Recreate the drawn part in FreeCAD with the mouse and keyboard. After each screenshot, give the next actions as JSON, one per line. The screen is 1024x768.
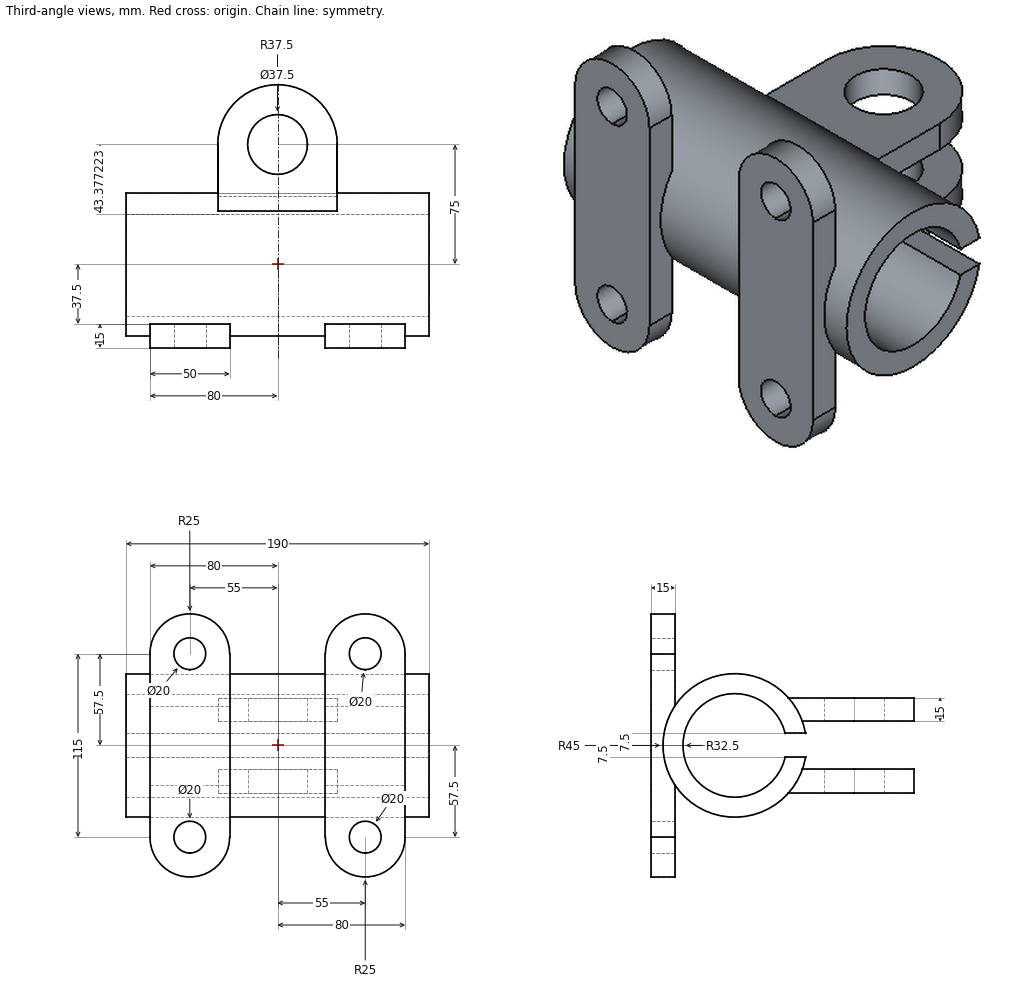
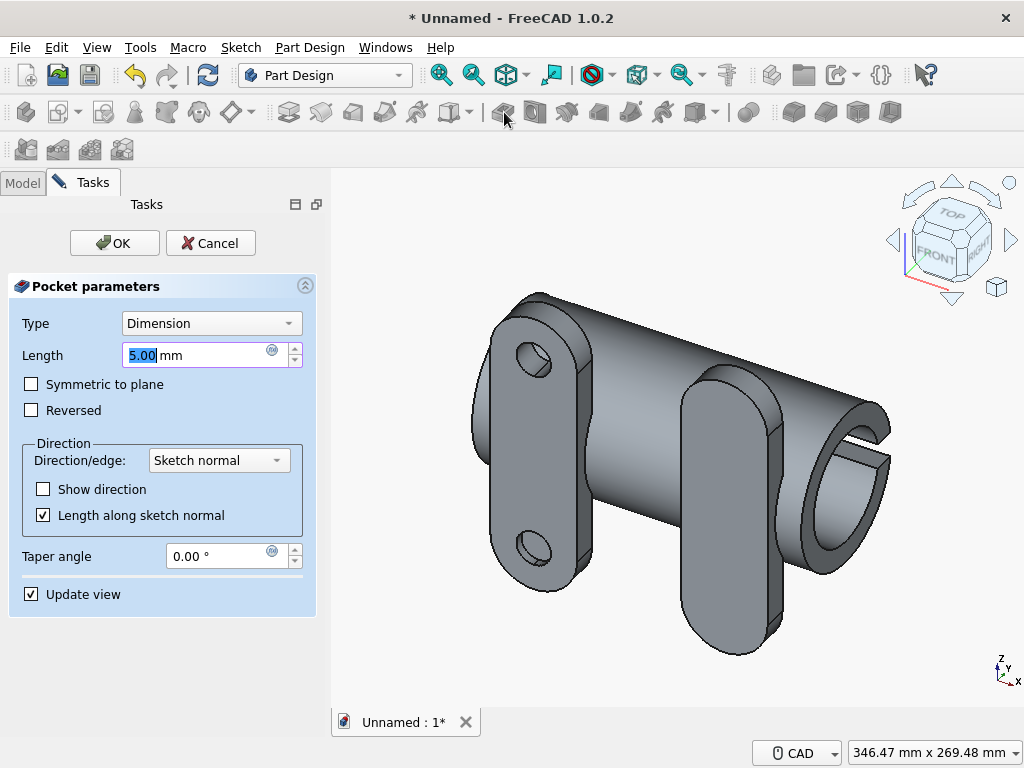
{"action": "left_click", "coordinate": [212, 324]}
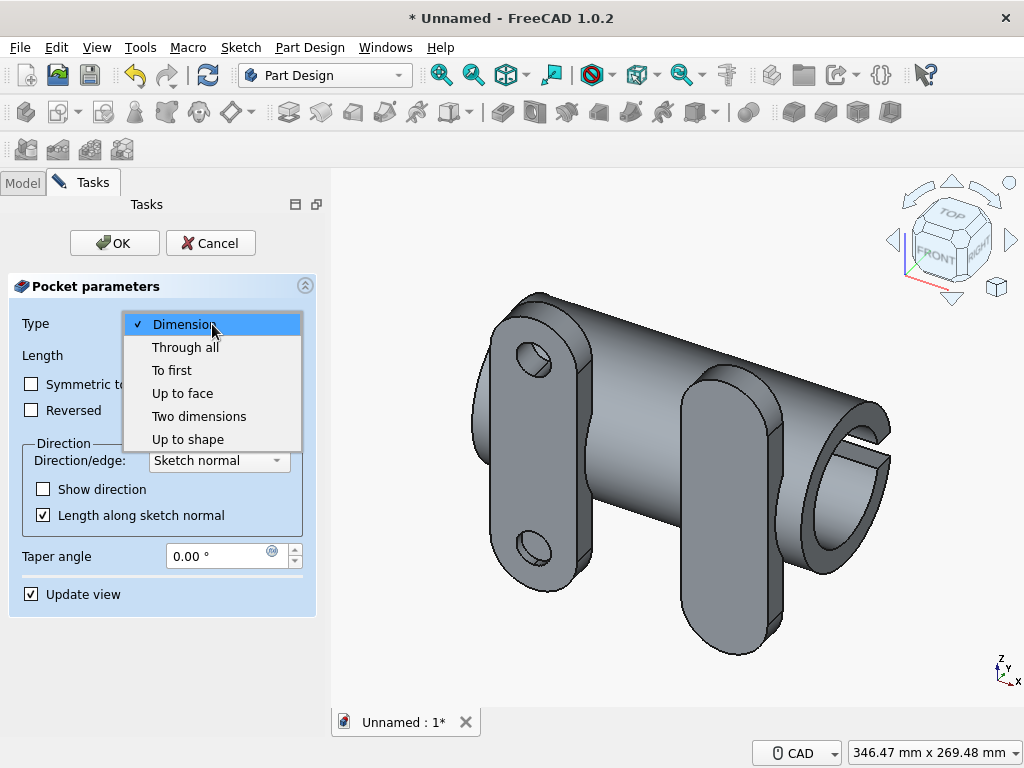
{"action": "left_click", "coordinate": [212, 370]}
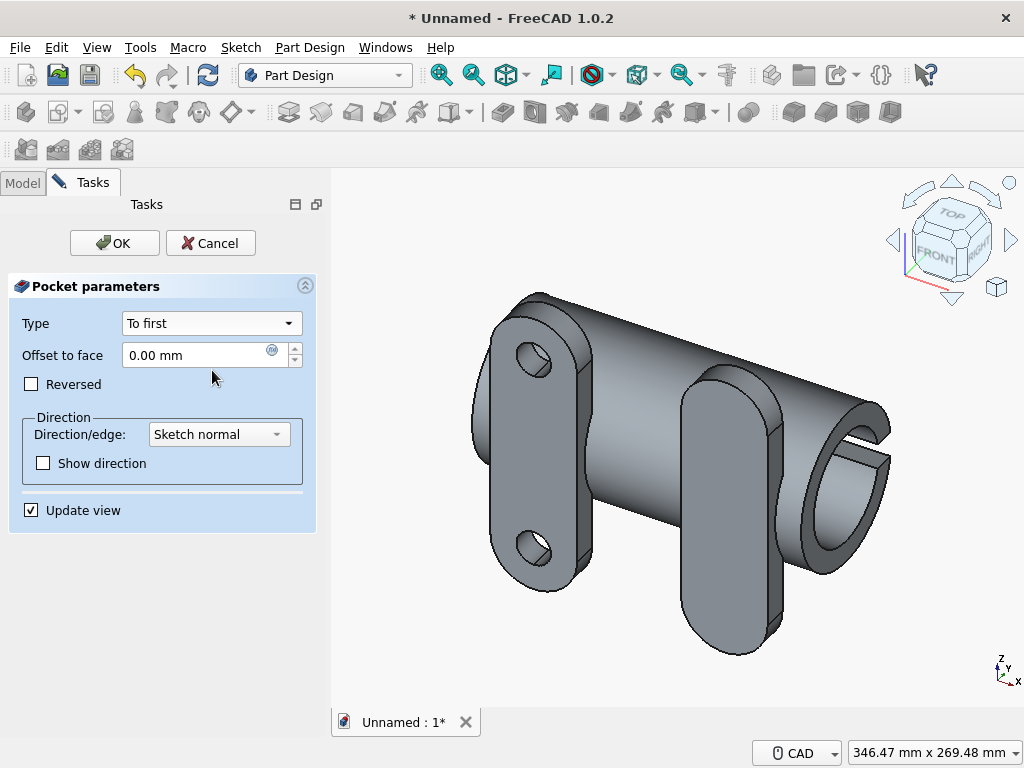
{"action": "left_click", "coordinate": [115, 243]}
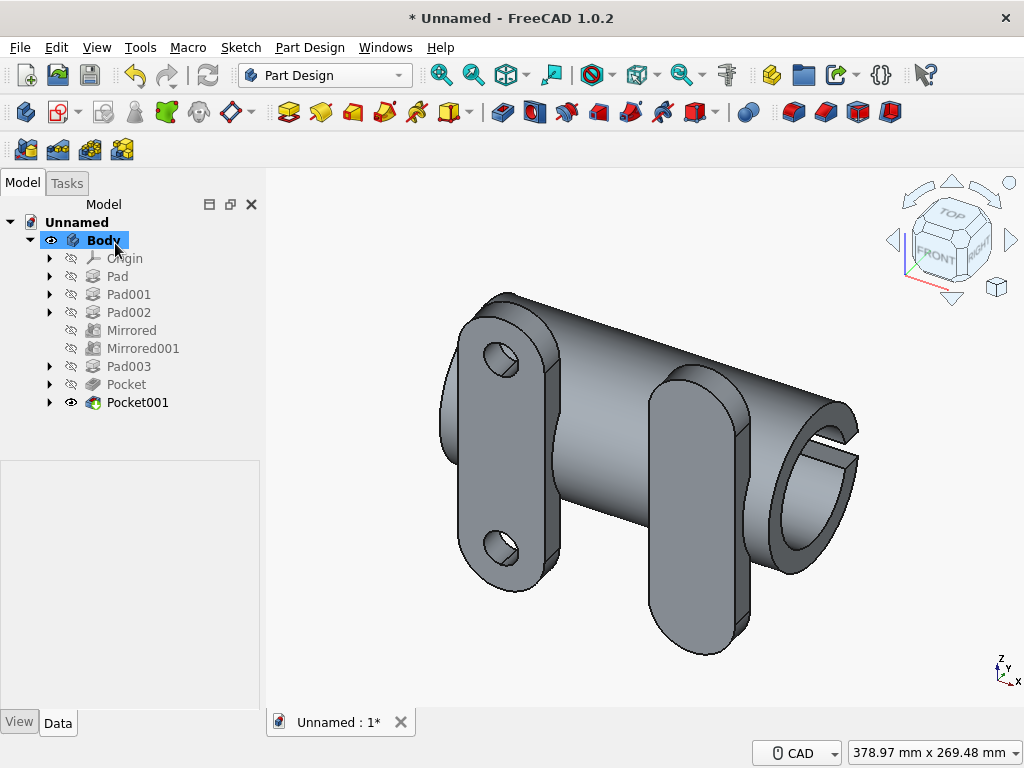
{"action": "left_click", "coordinate": [692, 516]}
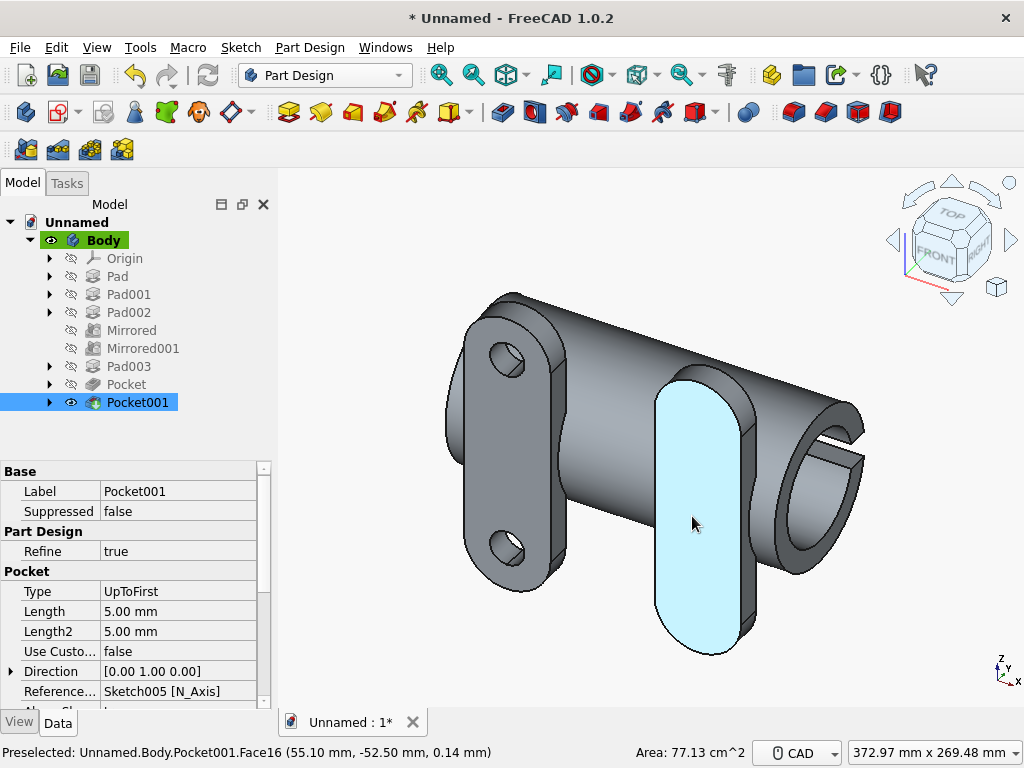
{"action": "left_click", "coordinate": [58, 112]}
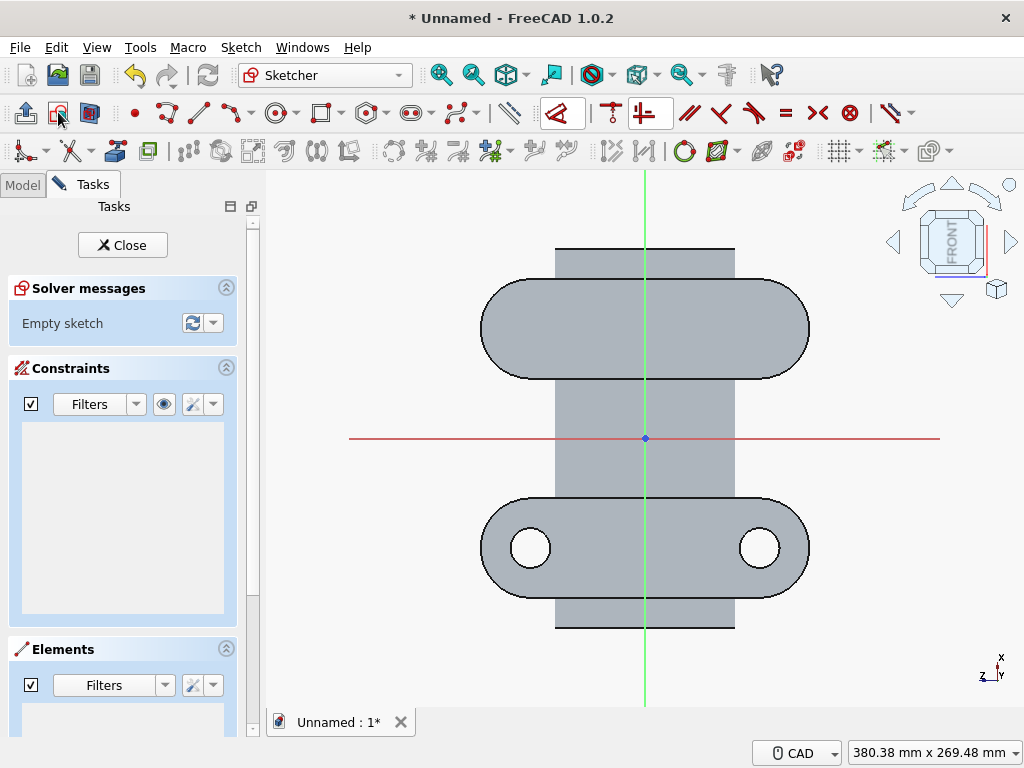
{"action": "scroll", "coordinate": [782, 315], "scroll_direction": "up", "scroll_amount": 11}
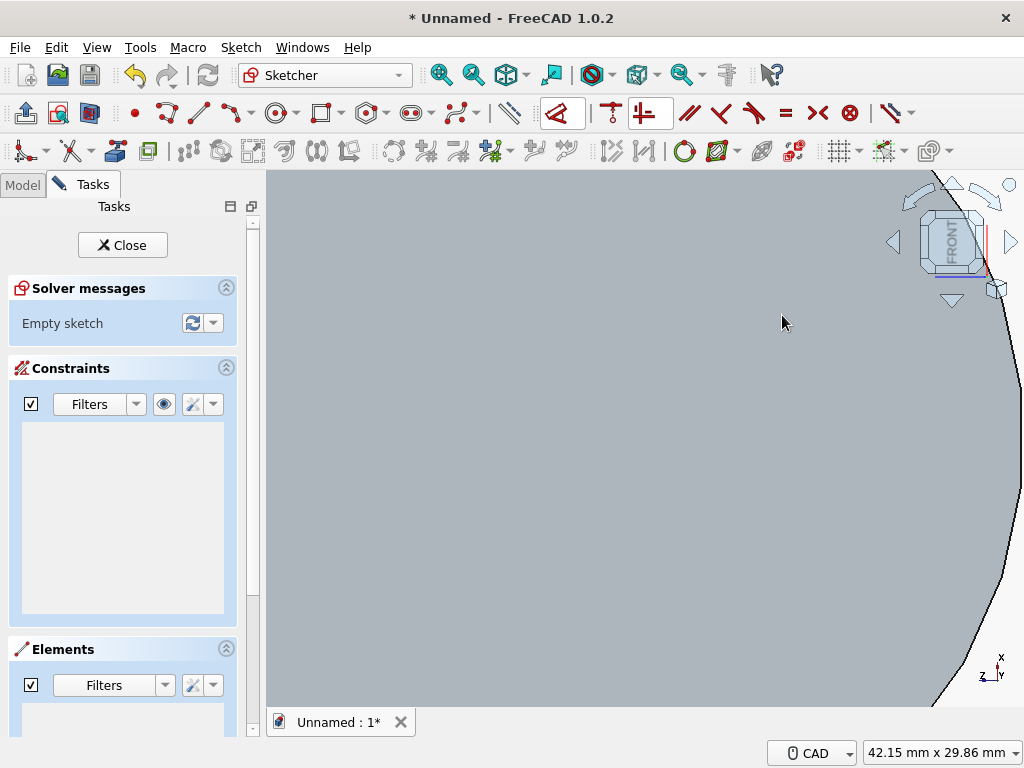
{"action": "left_click", "coordinate": [276, 114]}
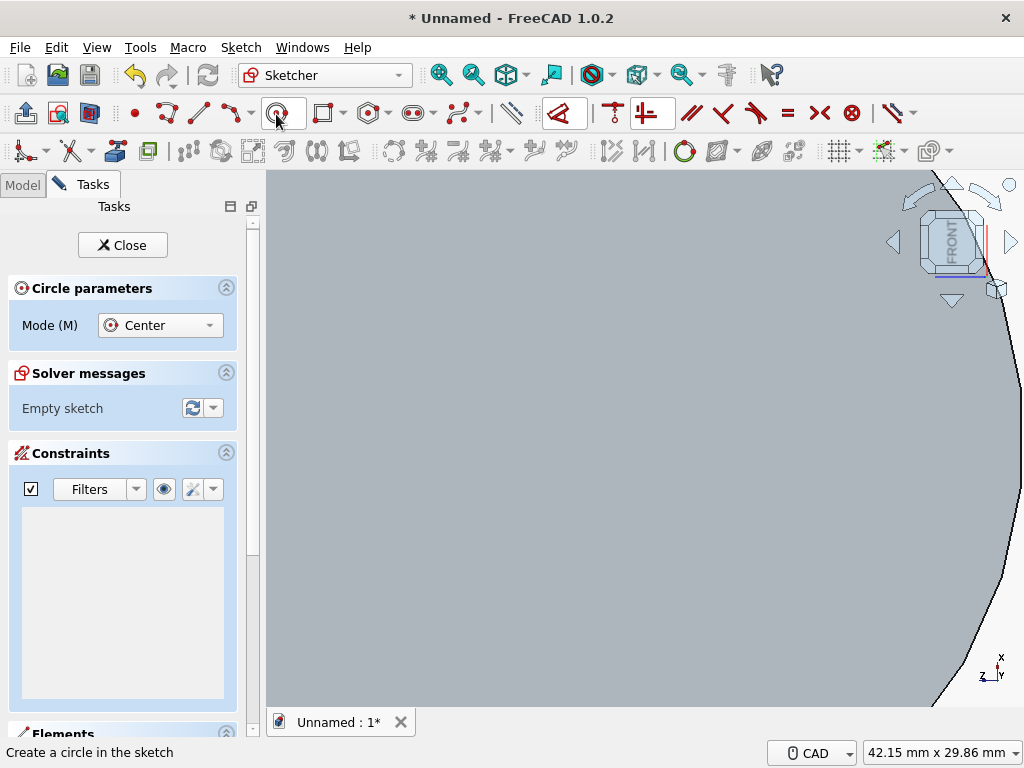
{"action": "left_click", "coordinate": [574, 438]}
{"action": "left_click", "coordinate": [701, 311]}
{"action": "key", "text": "Escape"}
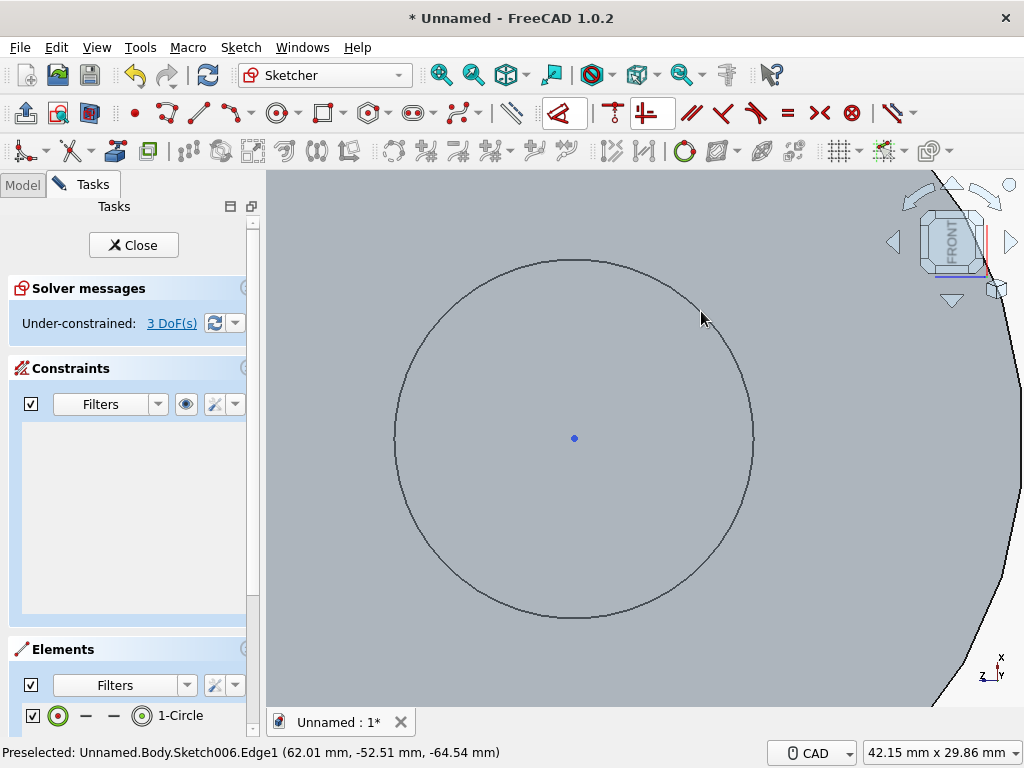
{"action": "left_click", "coordinate": [701, 312]}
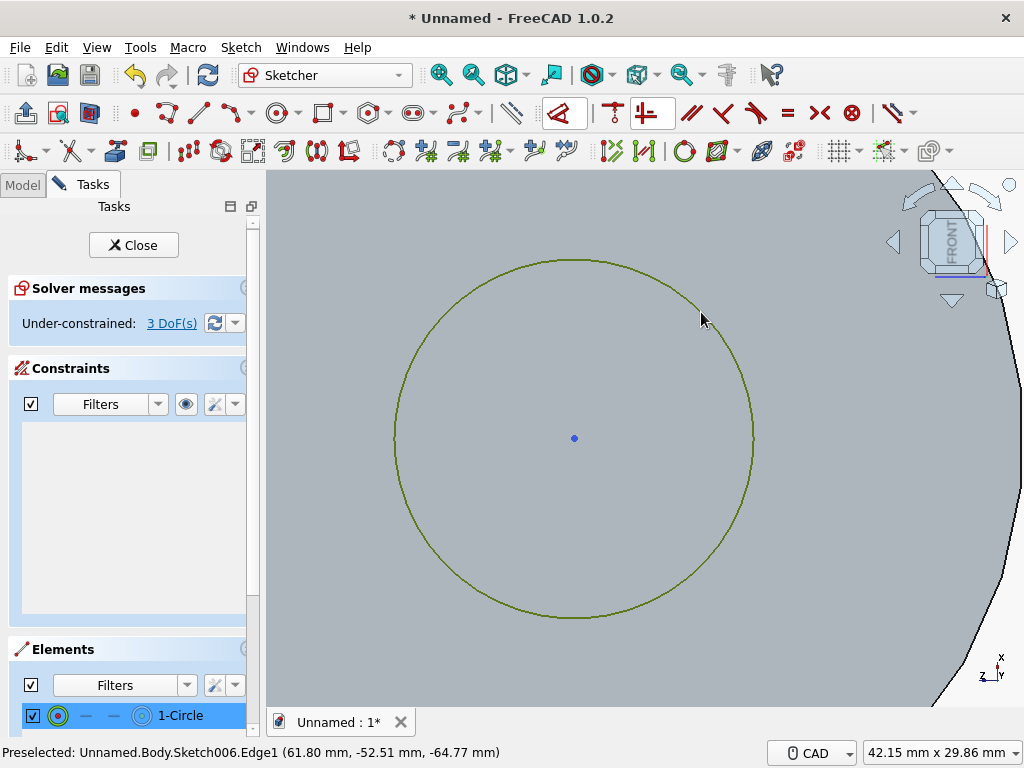
{"action": "left_click", "coordinate": [582, 114]}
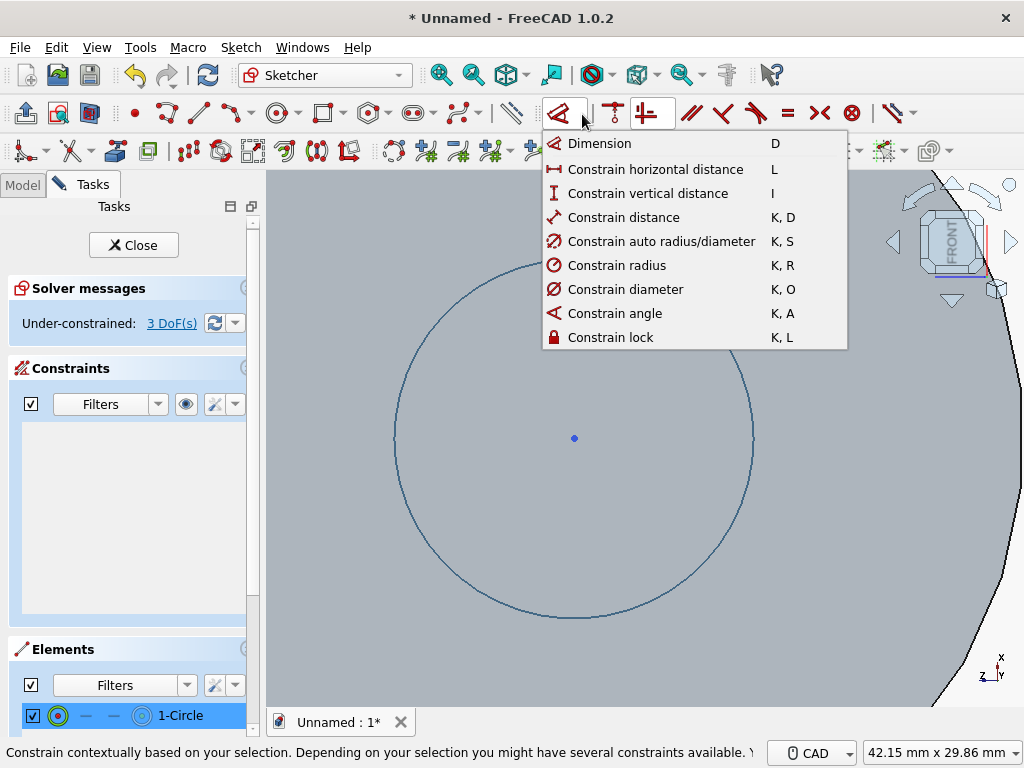
{"action": "left_click", "coordinate": [695, 289]}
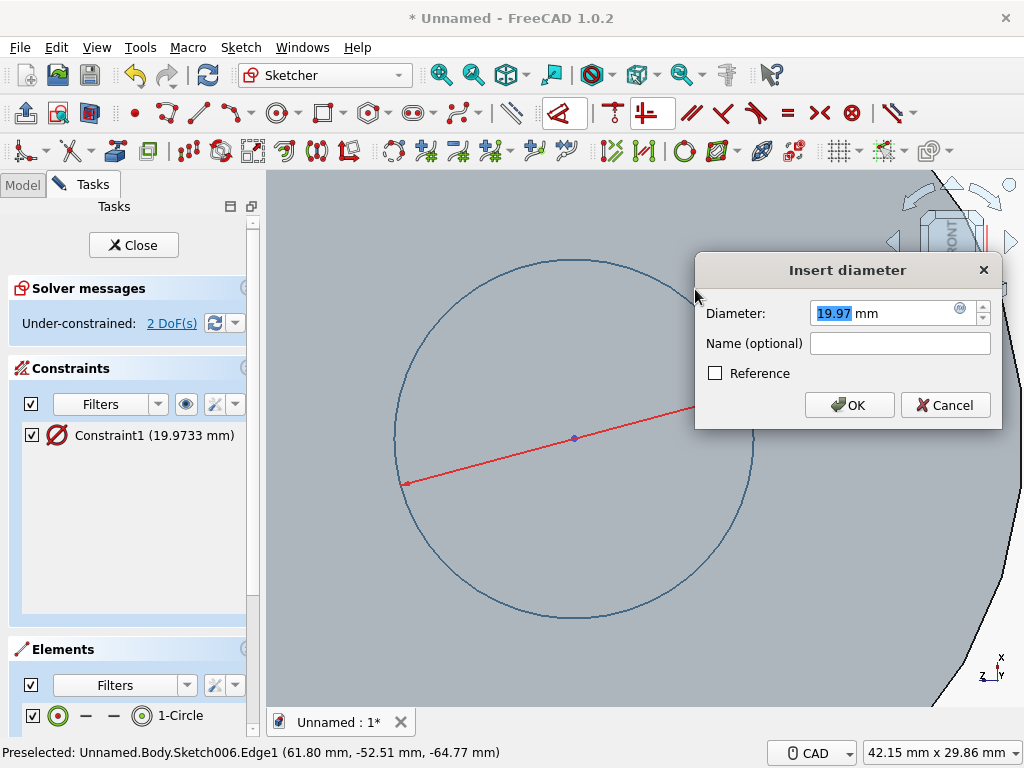
{"action": "type", "text": "20"}
{"action": "key", "text": "Return"}